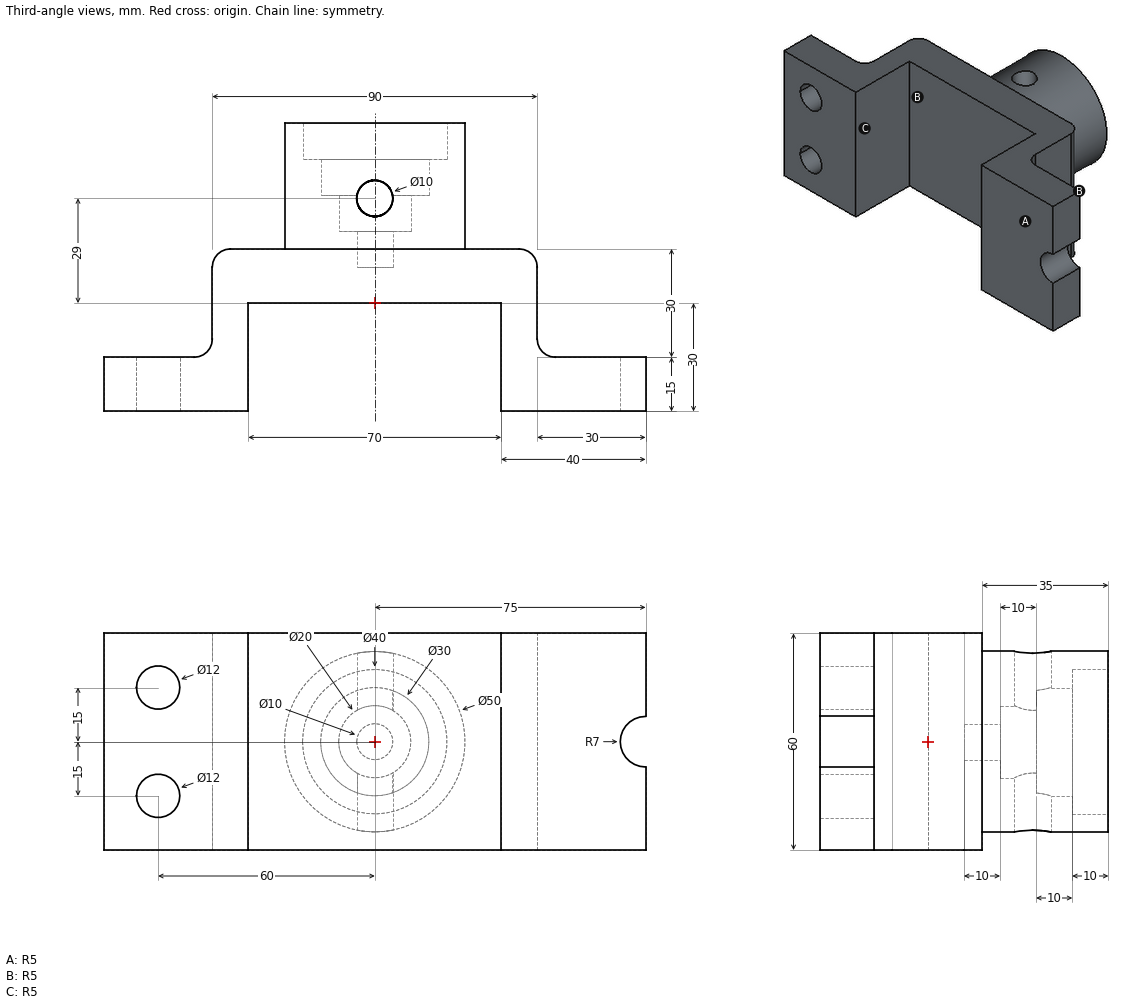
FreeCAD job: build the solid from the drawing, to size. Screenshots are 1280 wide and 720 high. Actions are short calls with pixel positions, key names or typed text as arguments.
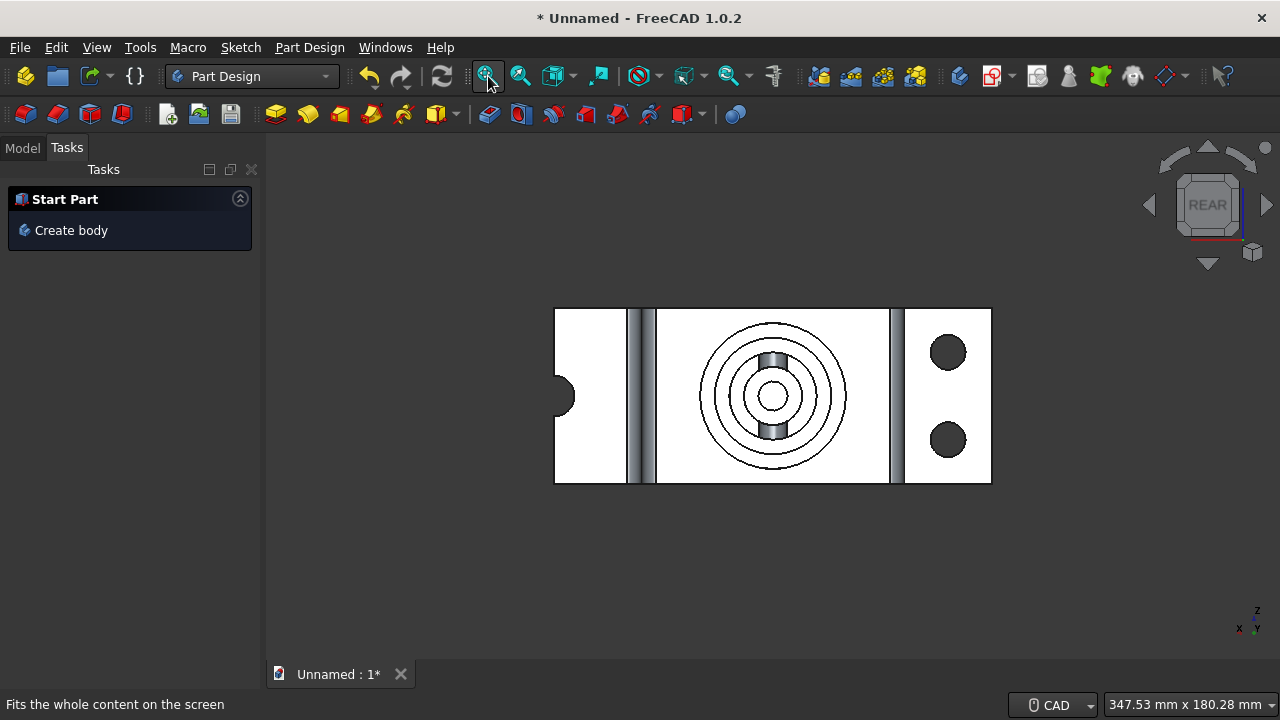
key(0)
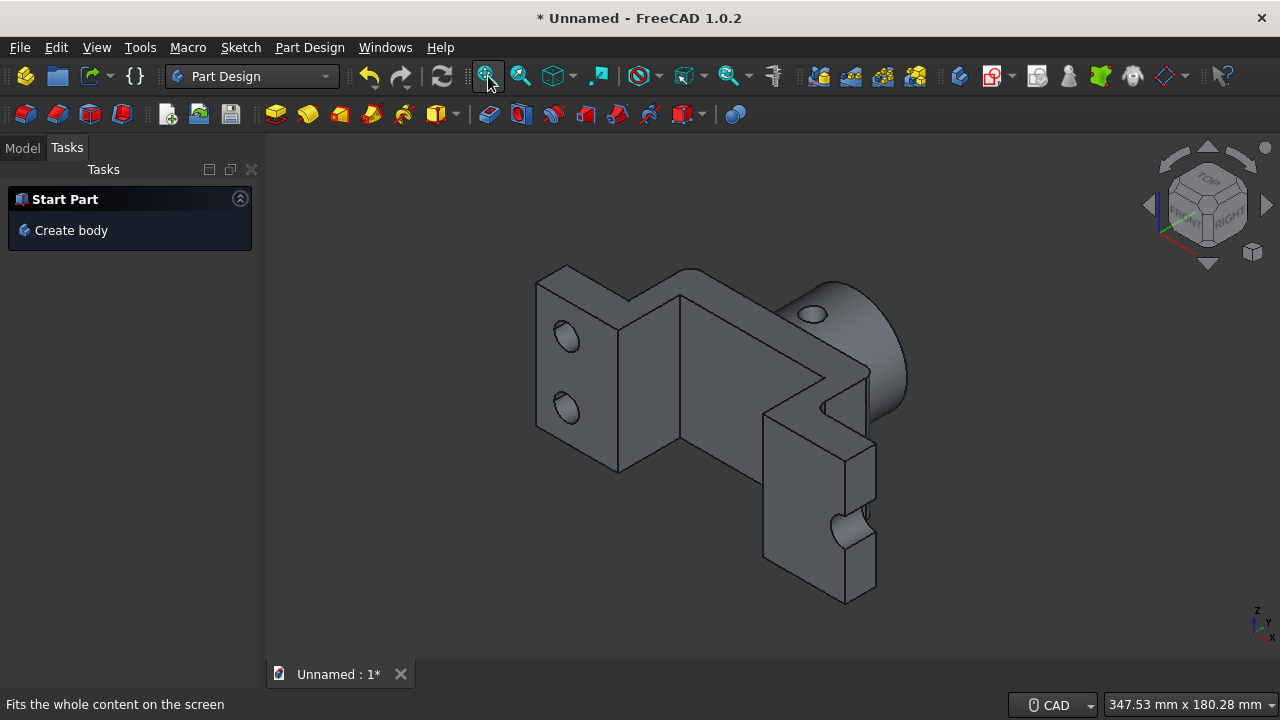
key(2)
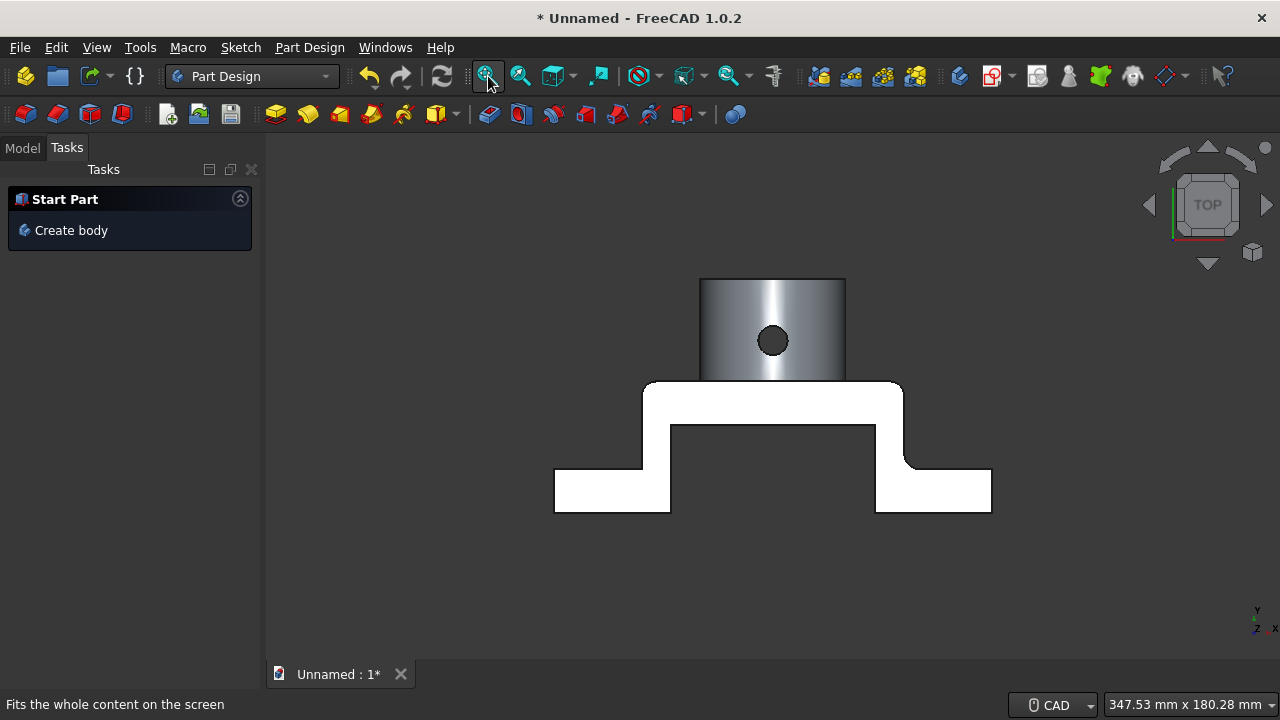
click(488, 76)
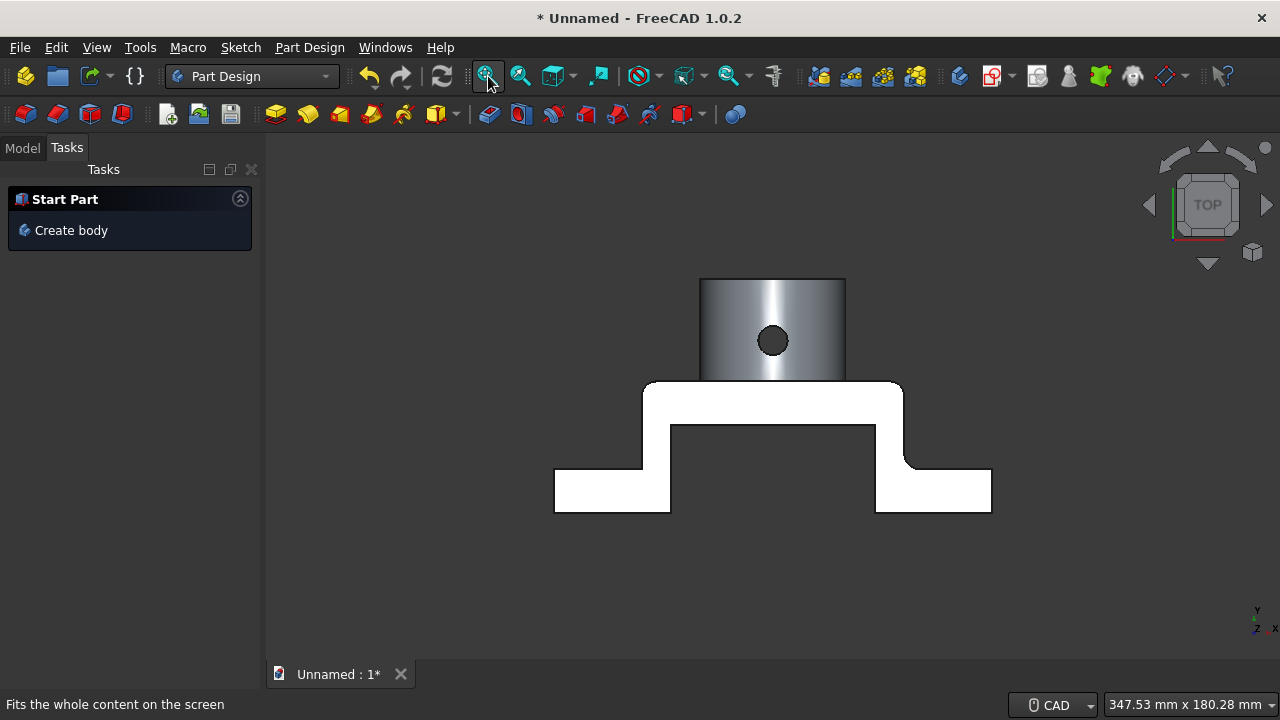
key(1)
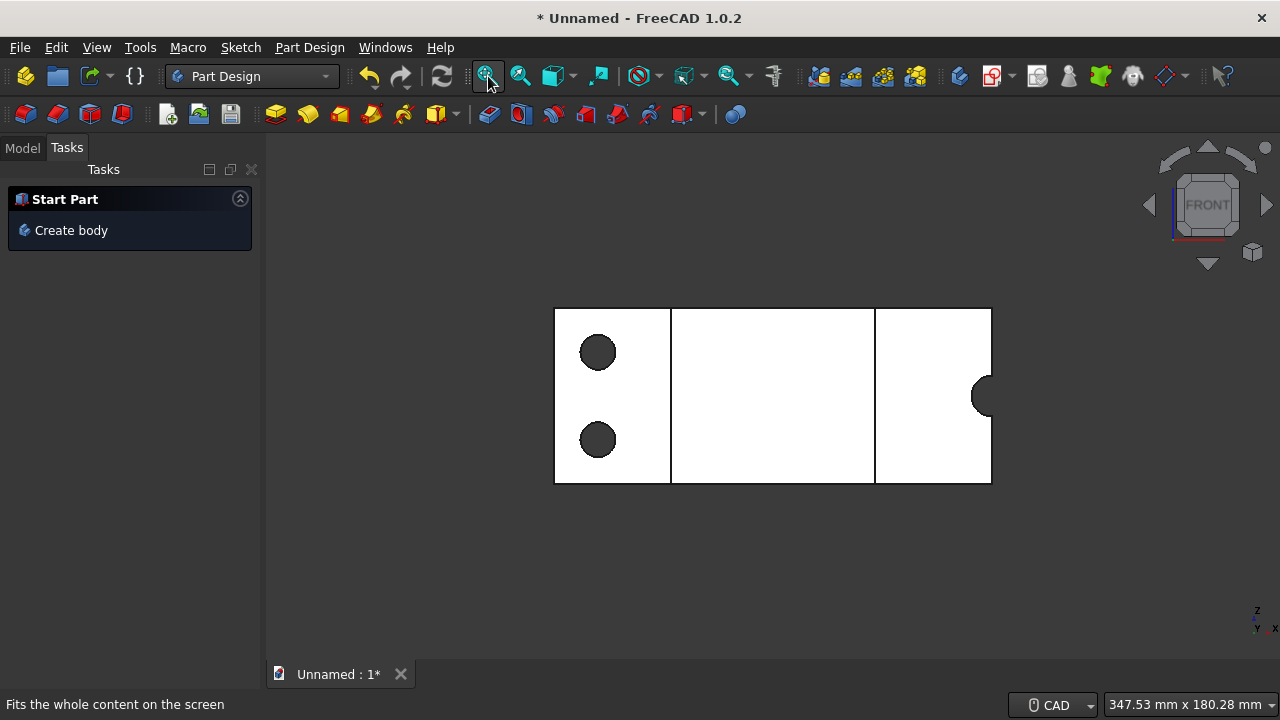
key(v)
key(f)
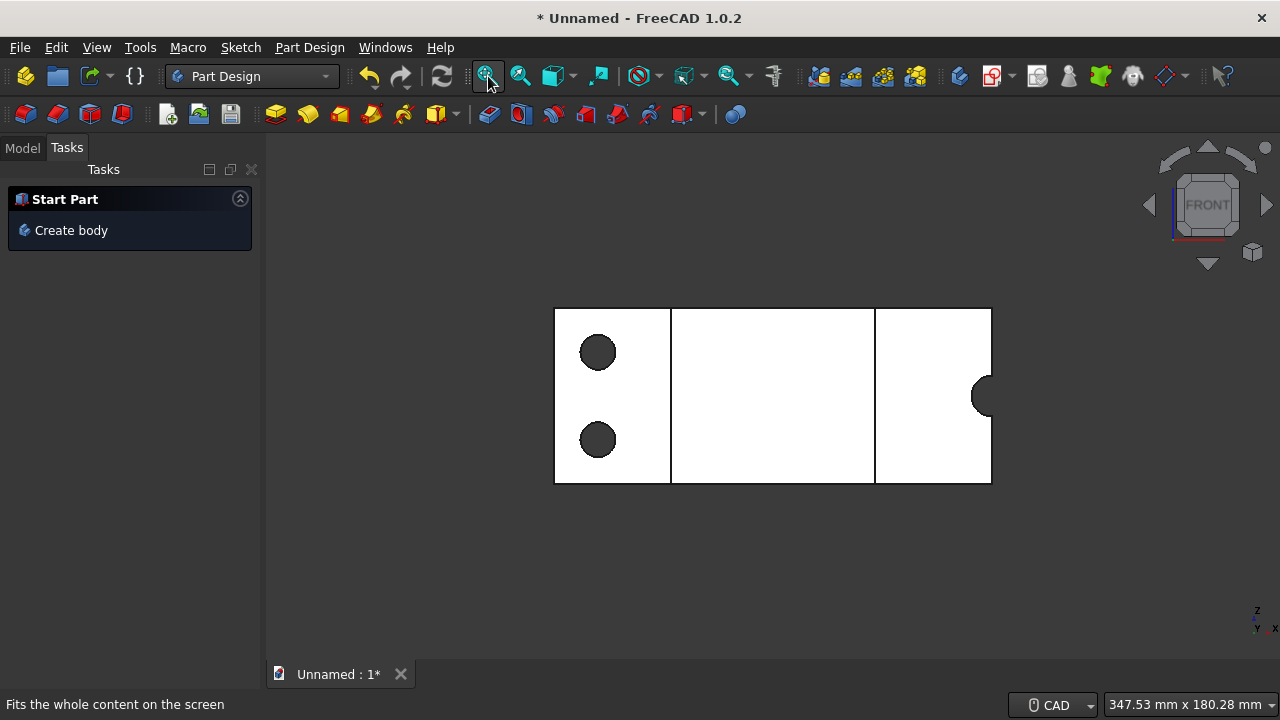
key(3)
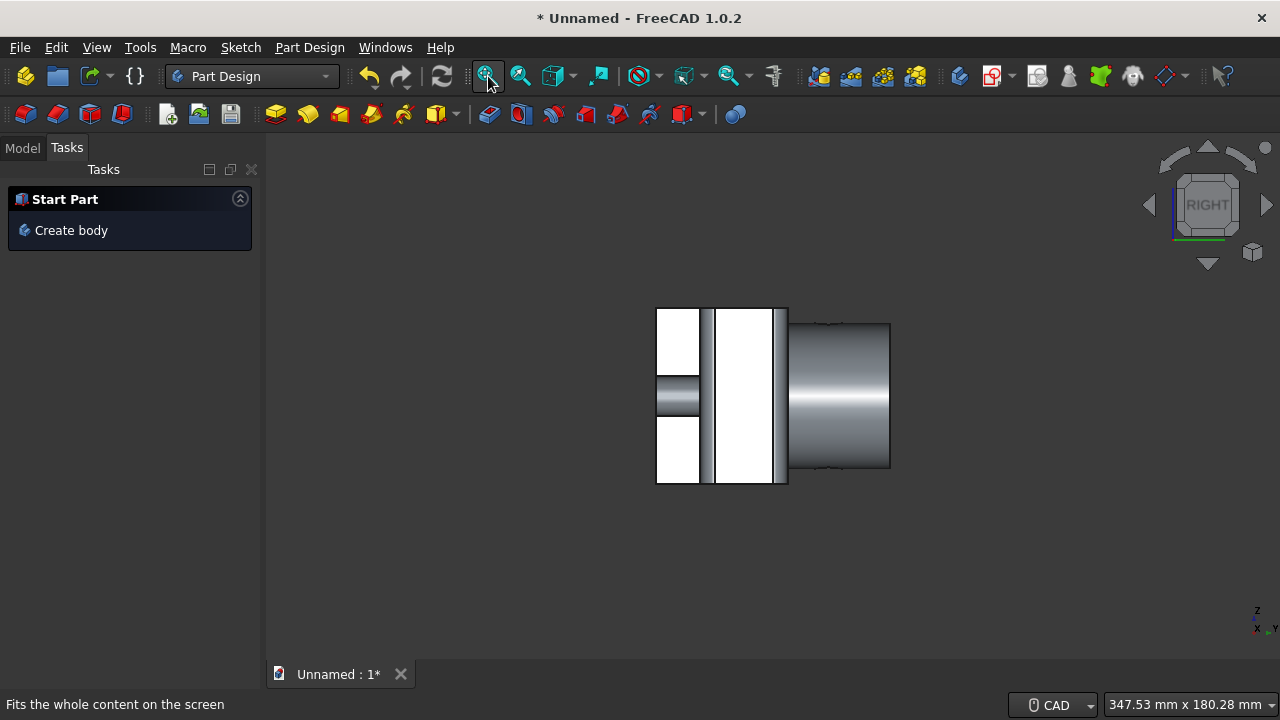
click(488, 76)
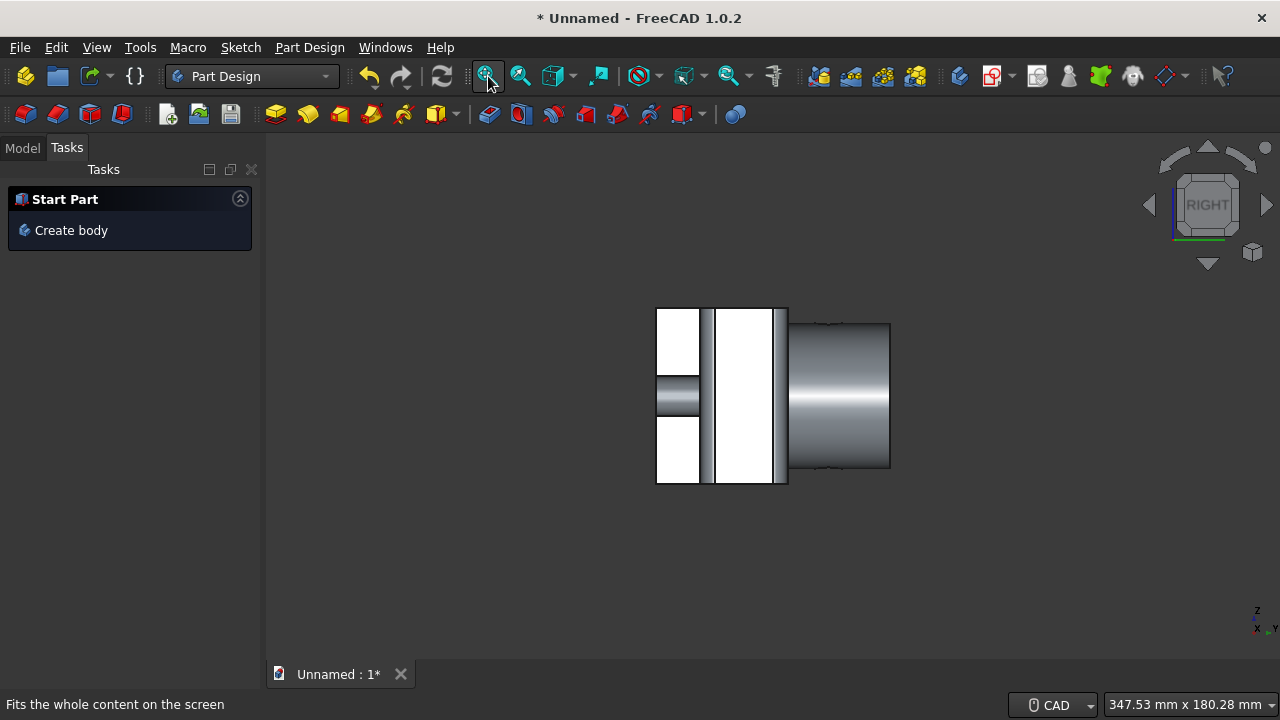
key(5)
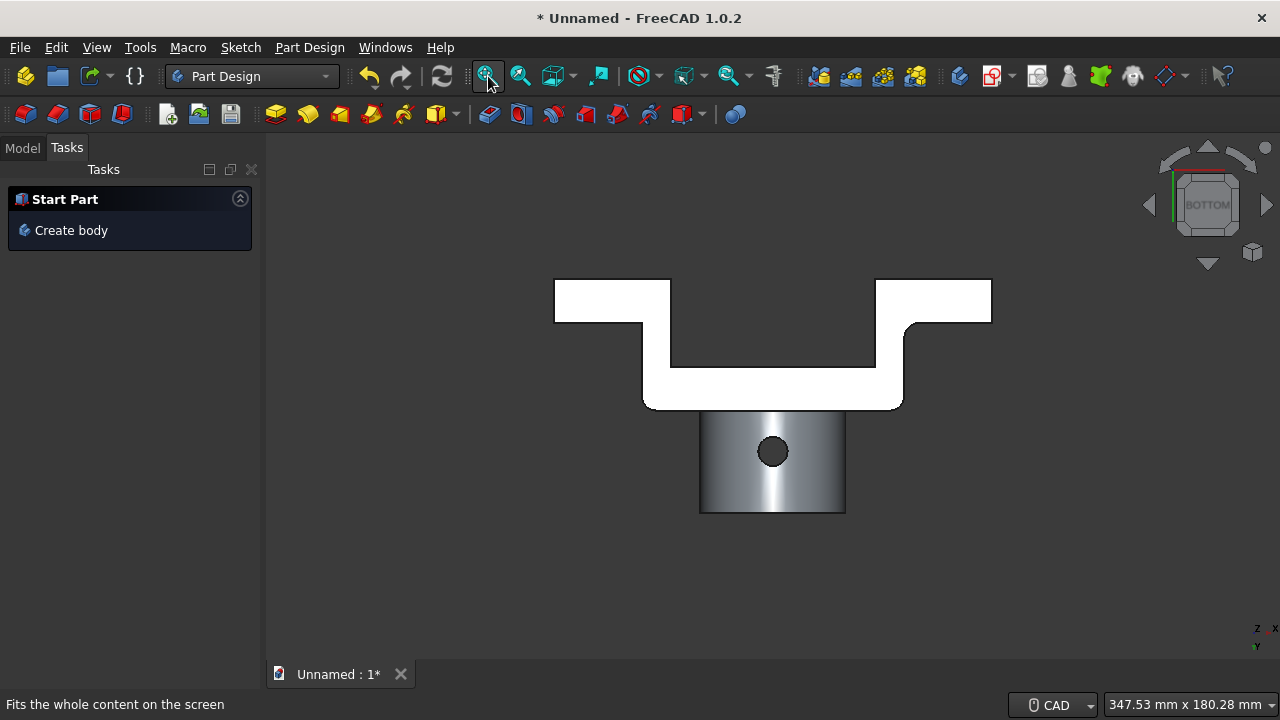
click(488, 76)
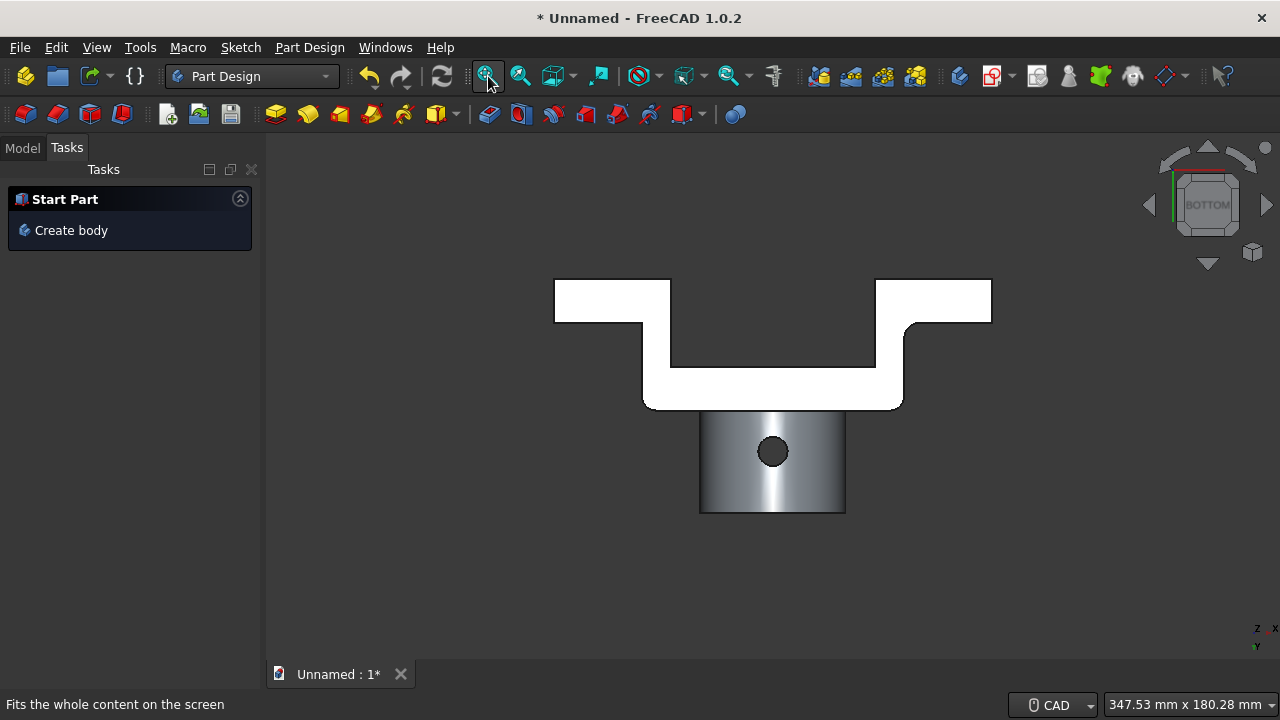
key(4)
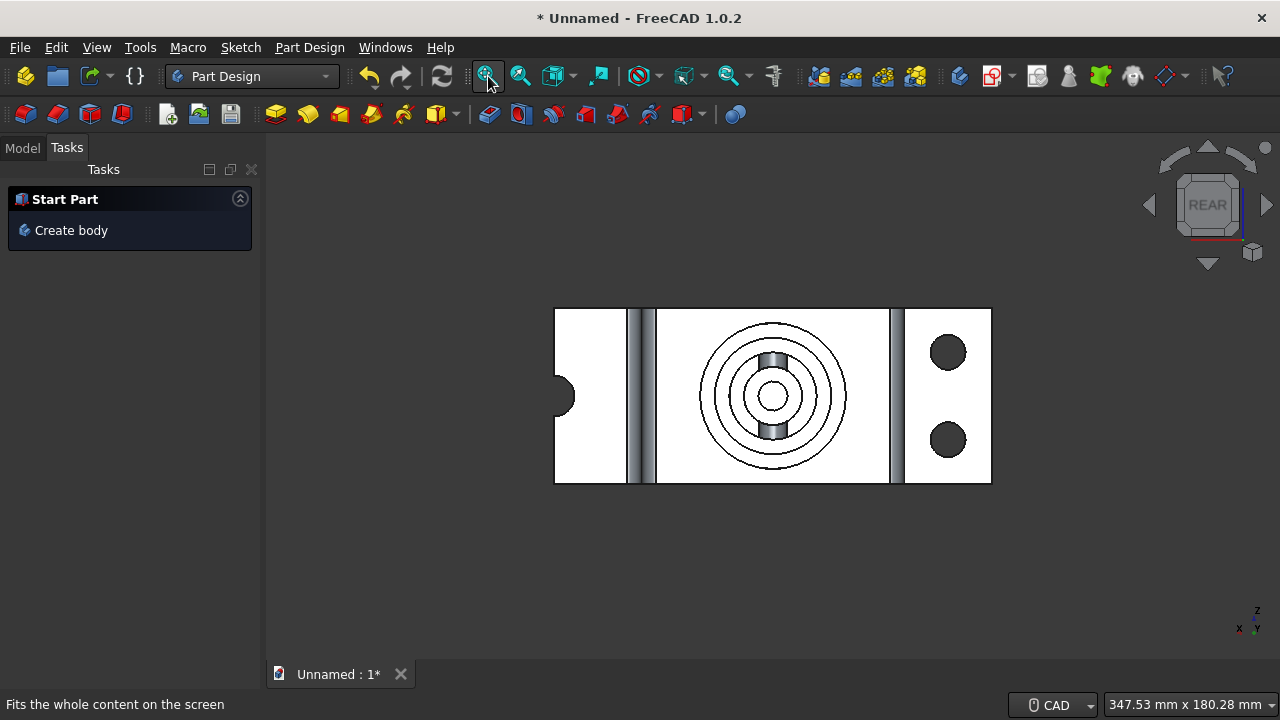
key(v)
key(f)